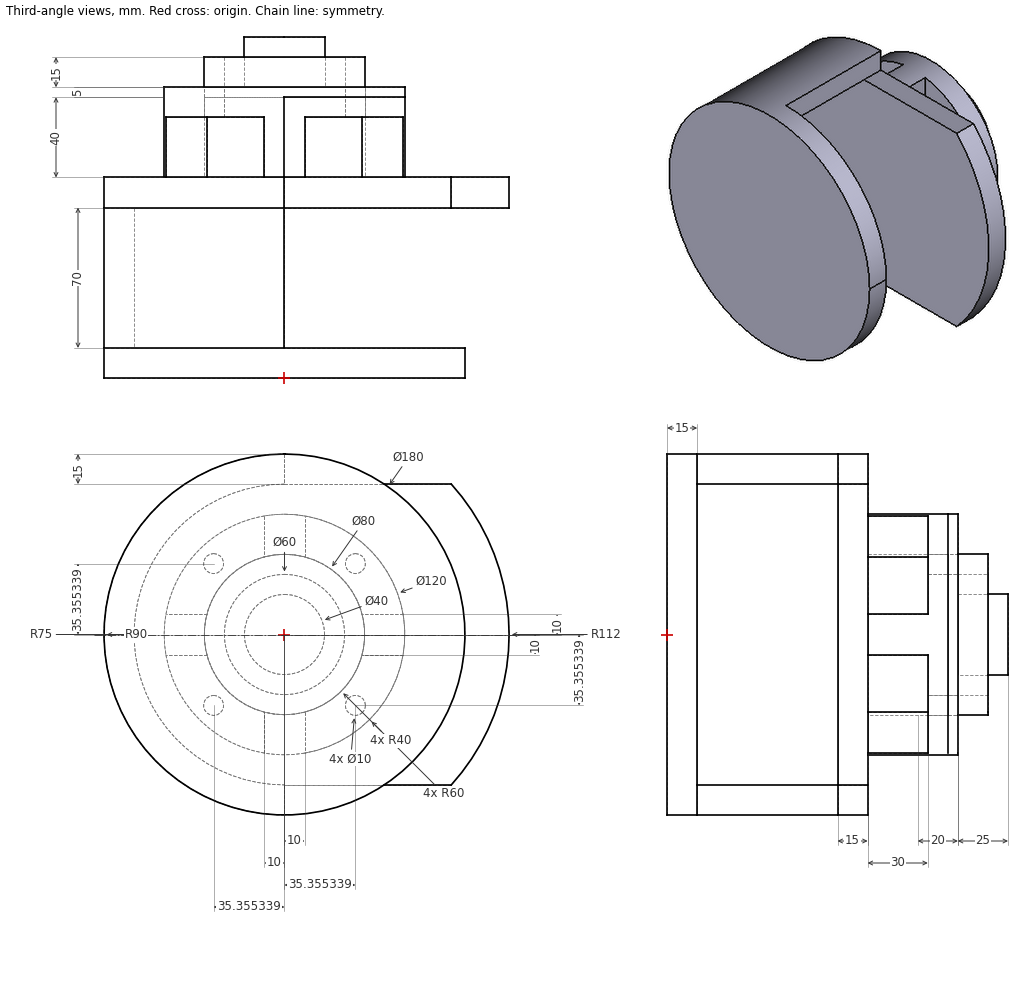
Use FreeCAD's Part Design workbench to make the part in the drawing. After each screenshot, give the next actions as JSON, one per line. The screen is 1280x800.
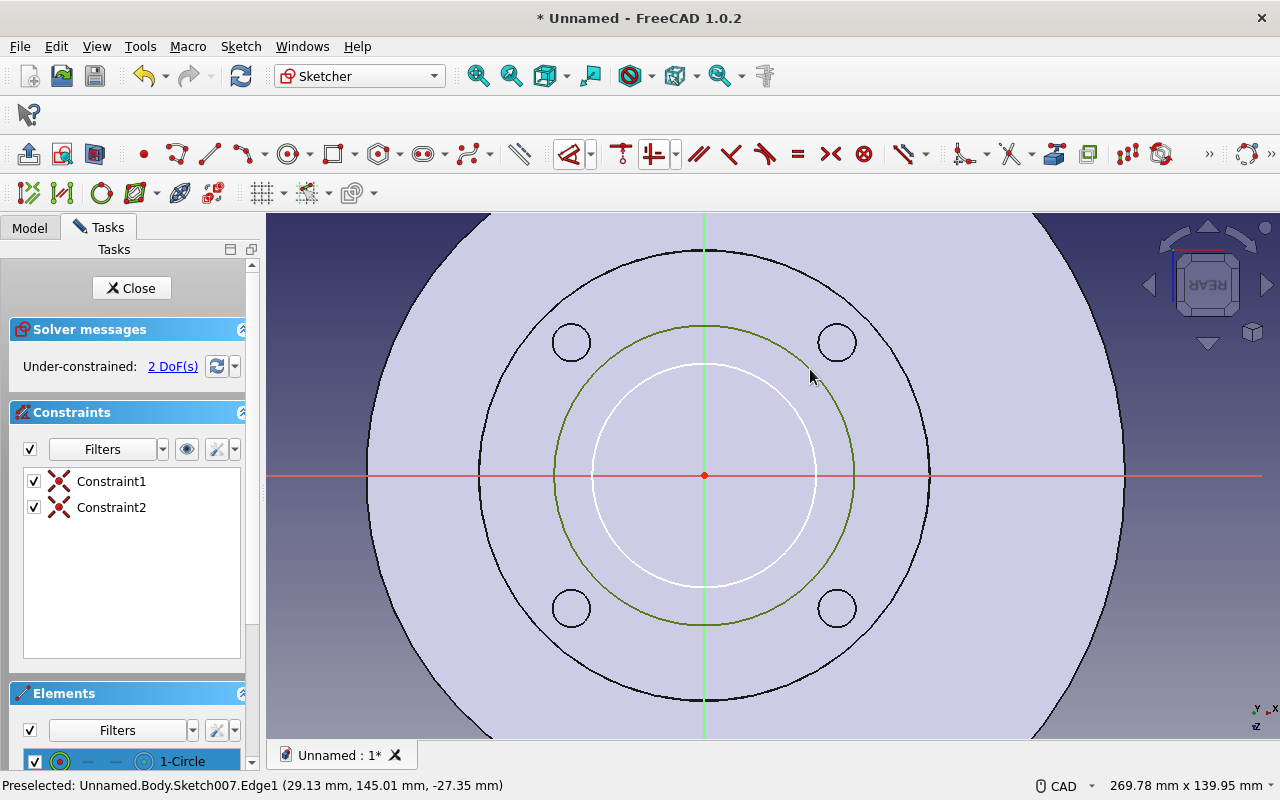
{"action": "key", "text": "k o"}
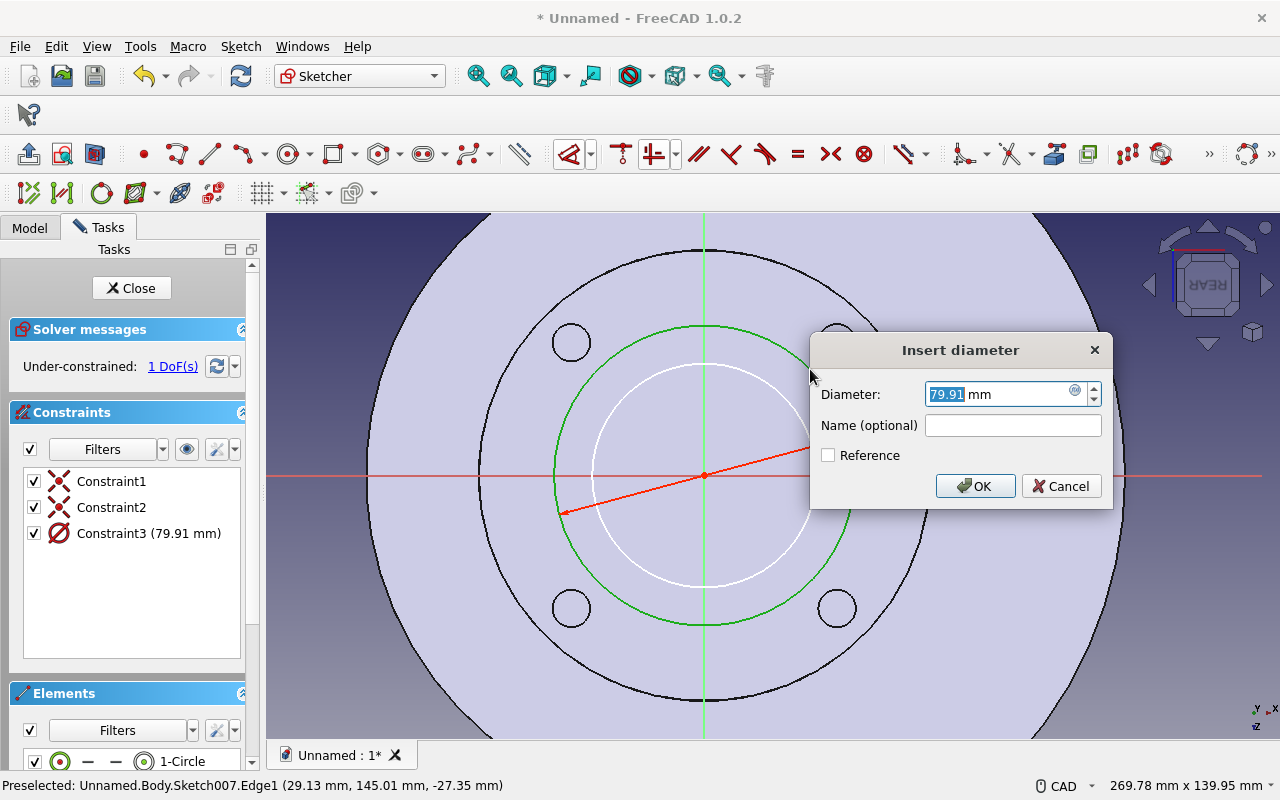
{"action": "type", "text": "80"}
{"action": "key", "text": "Return"}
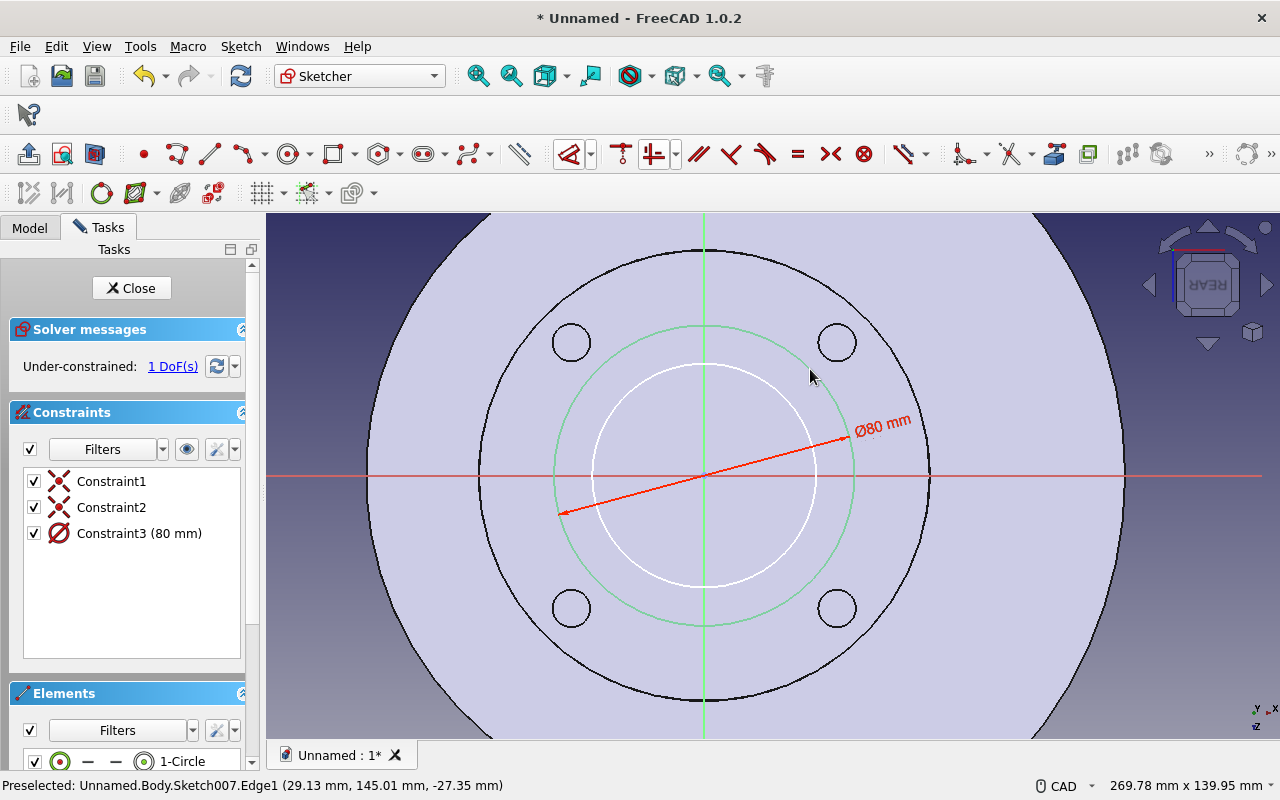
{"action": "left_click", "coordinate": [783, 396]}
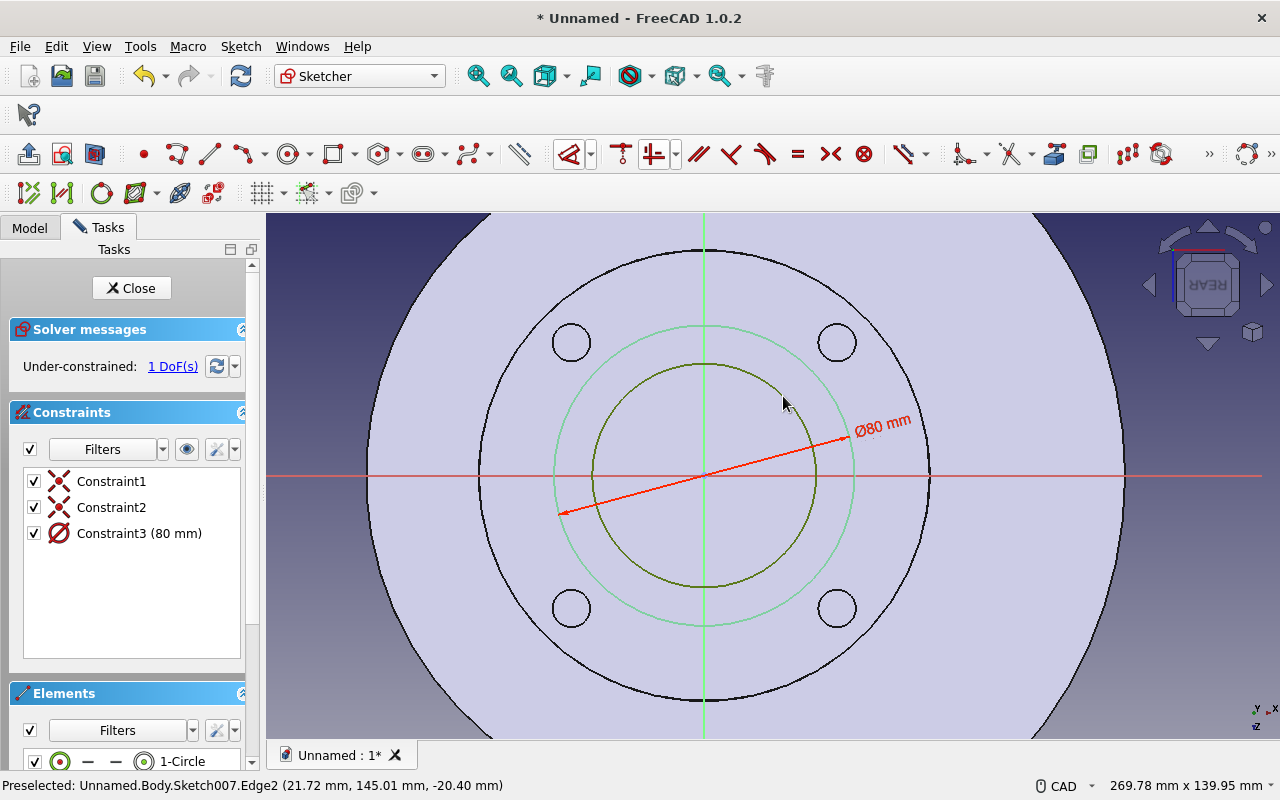
{"action": "key", "text": "k o"}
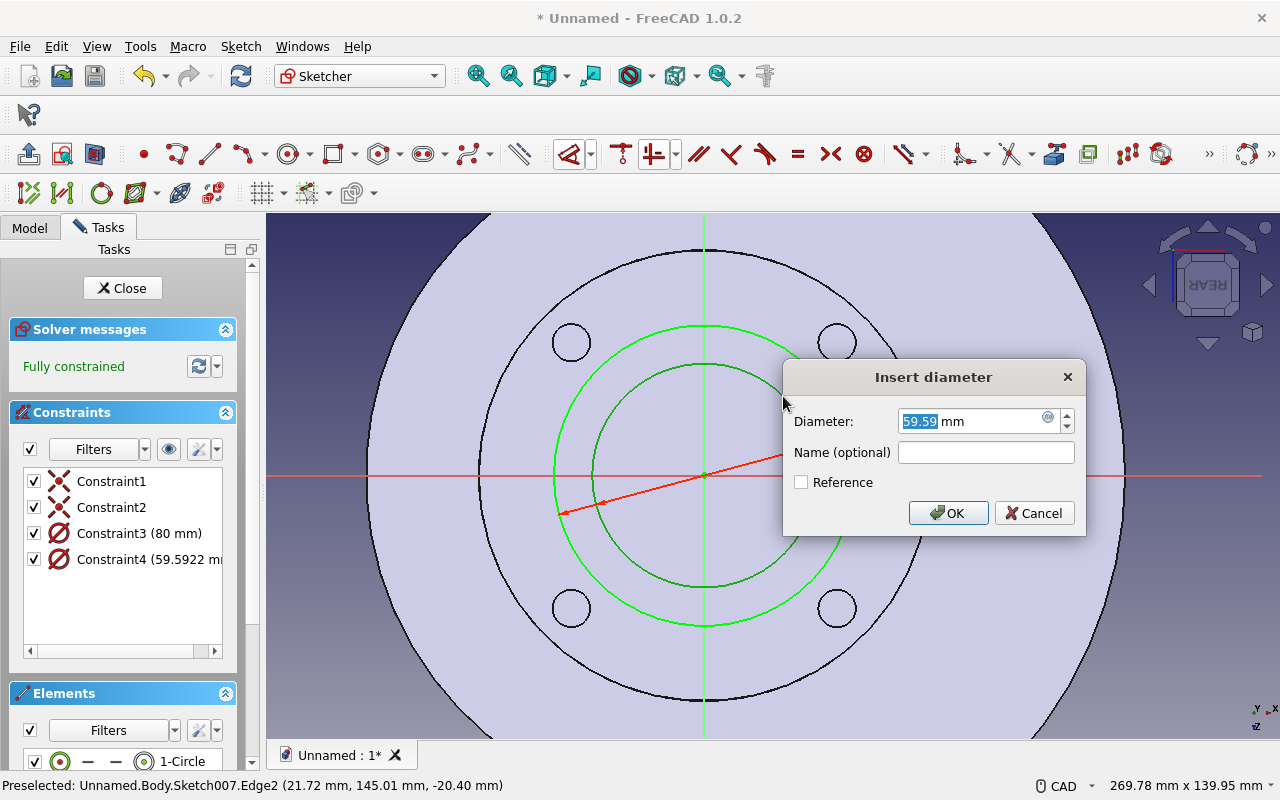
{"action": "type", "text": "60"}
{"action": "key", "text": "Return"}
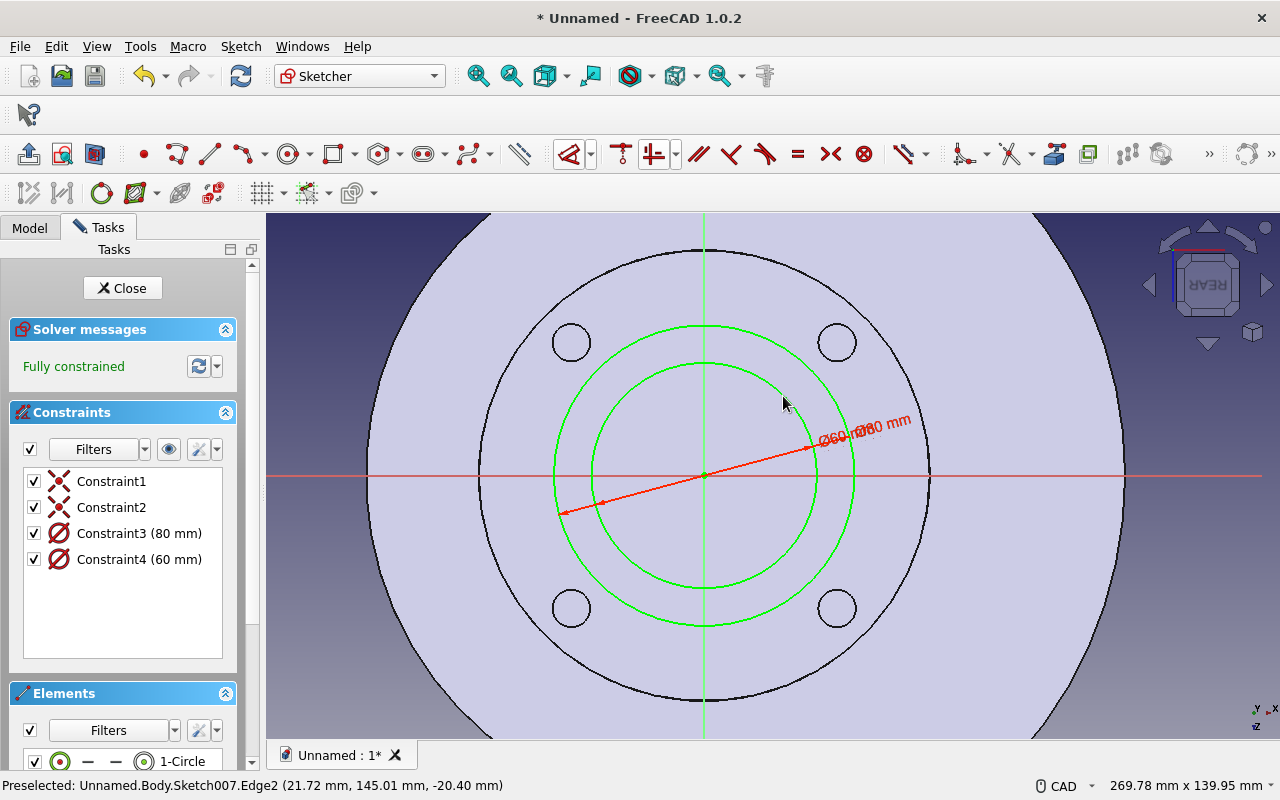
{"action": "left_click", "coordinate": [123, 288]}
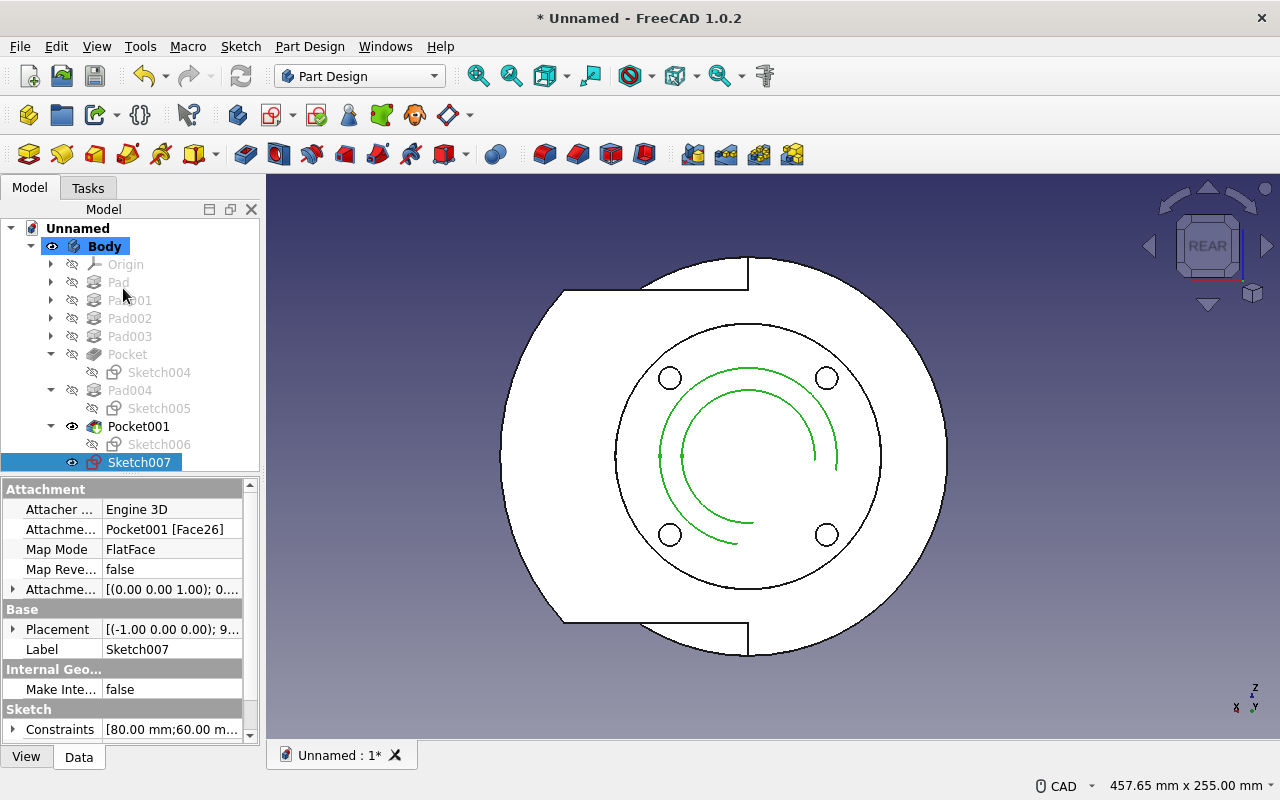
{"action": "left_click", "coordinate": [29, 154]}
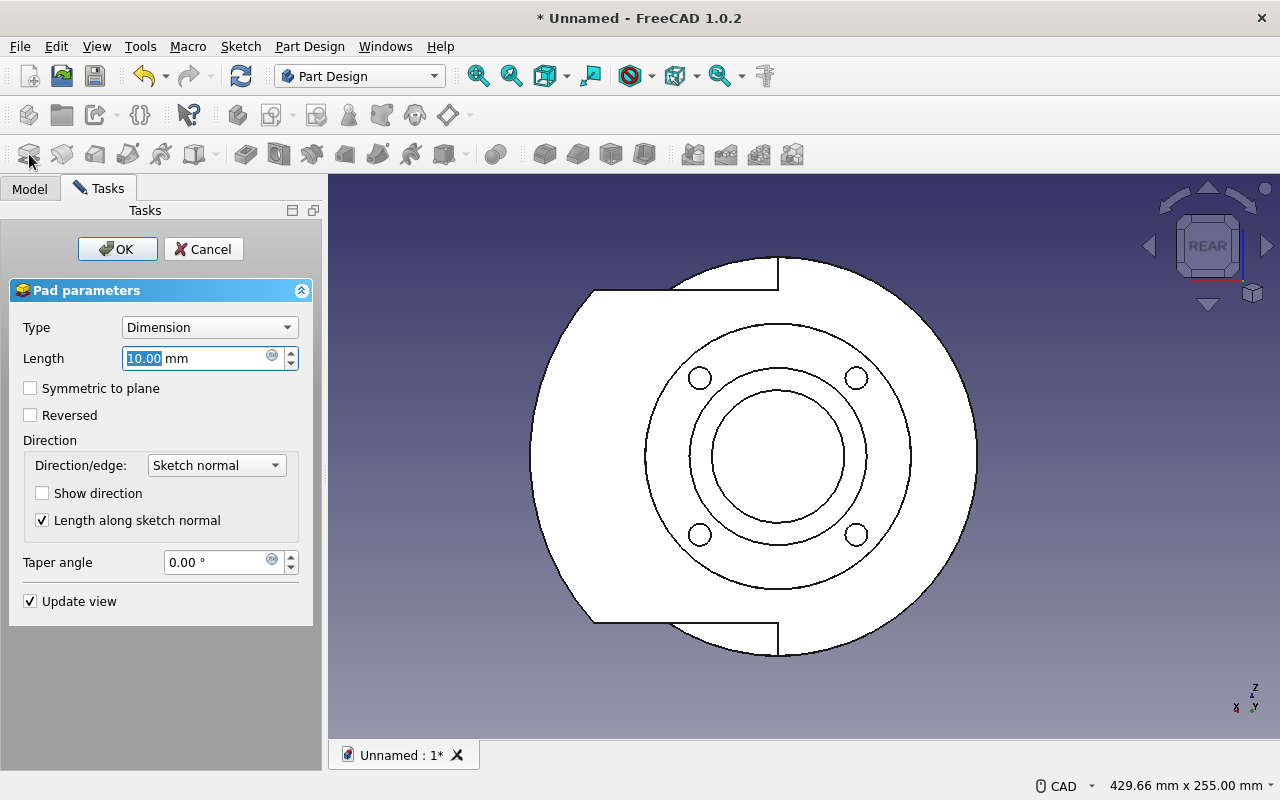
{"action": "type", "text": "15"}
{"action": "key", "text": "Tab"}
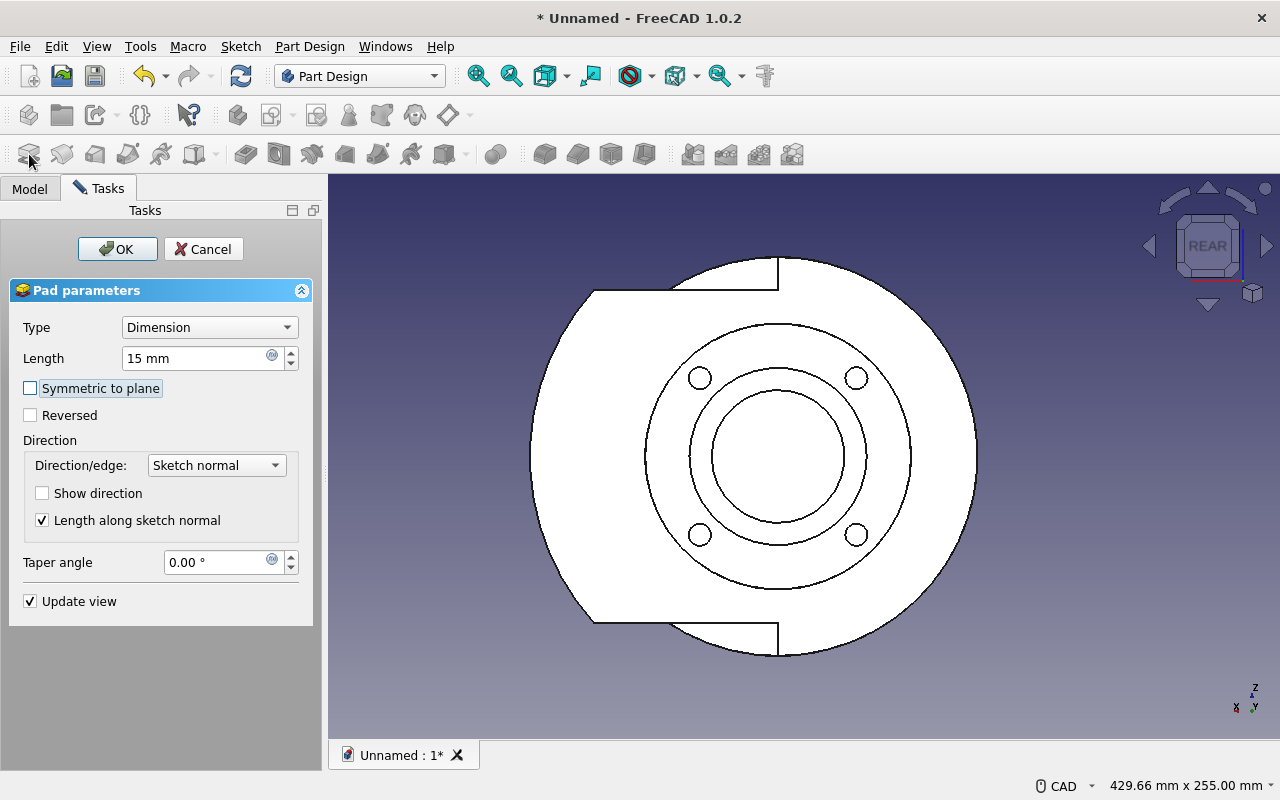
{"action": "left_click", "coordinate": [118, 249]}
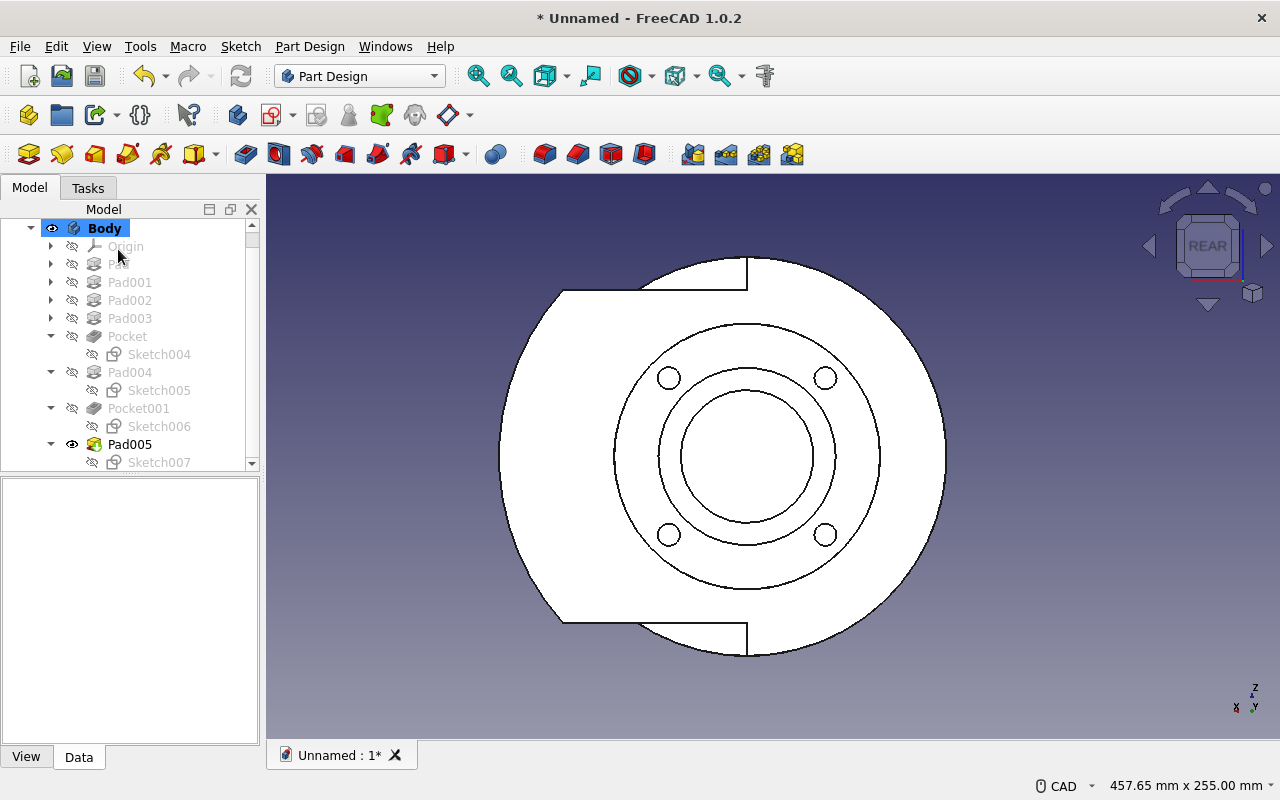
{"action": "left_click", "coordinate": [633, 455]}